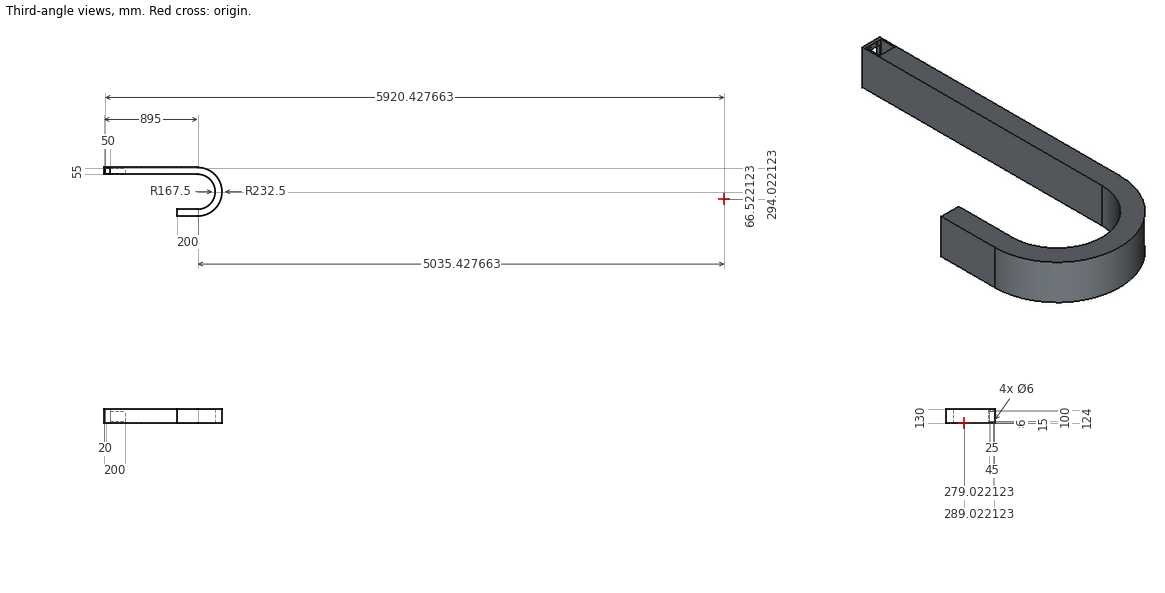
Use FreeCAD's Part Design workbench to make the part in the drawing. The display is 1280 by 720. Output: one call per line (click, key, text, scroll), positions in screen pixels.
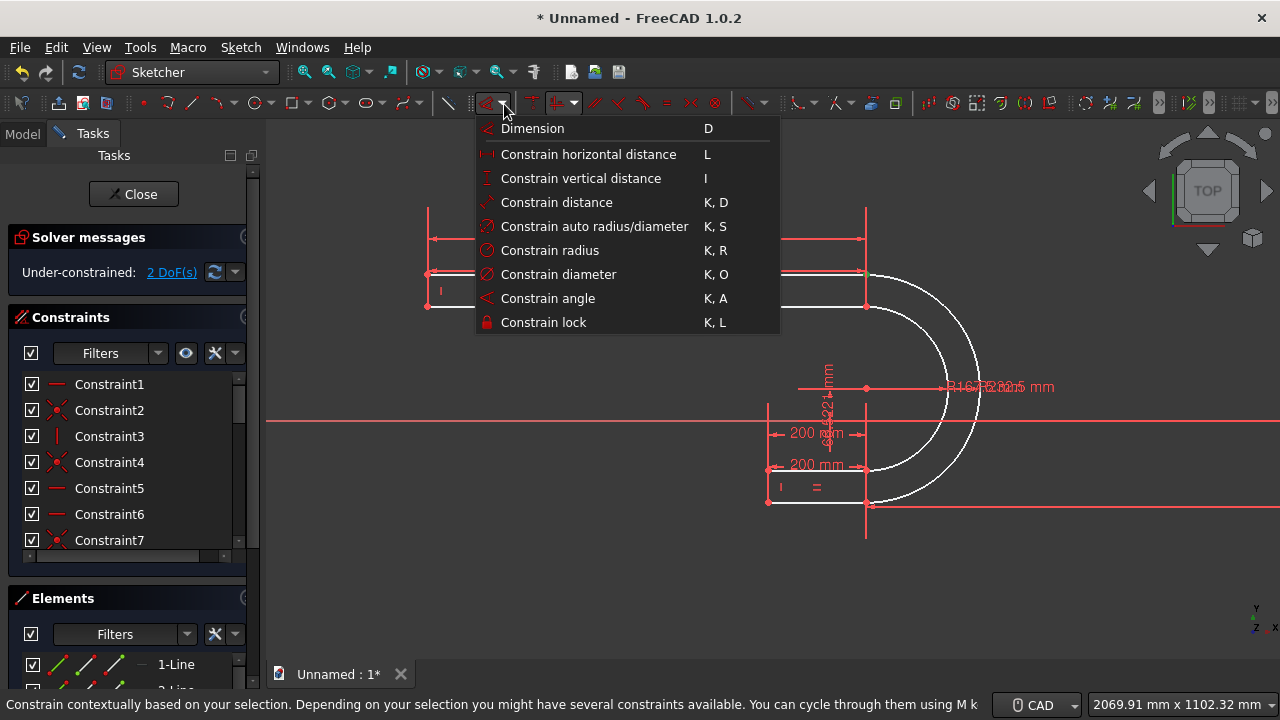
click(628, 154)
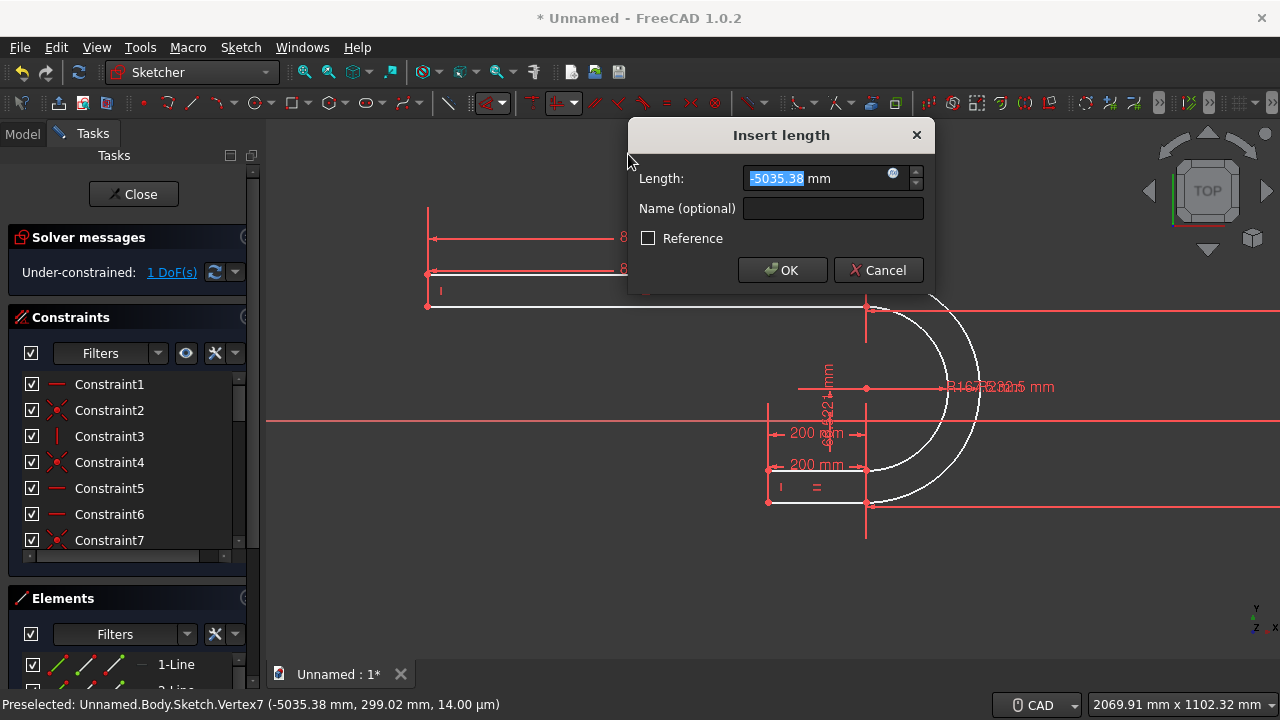
text(-5035.427663)
key(Return)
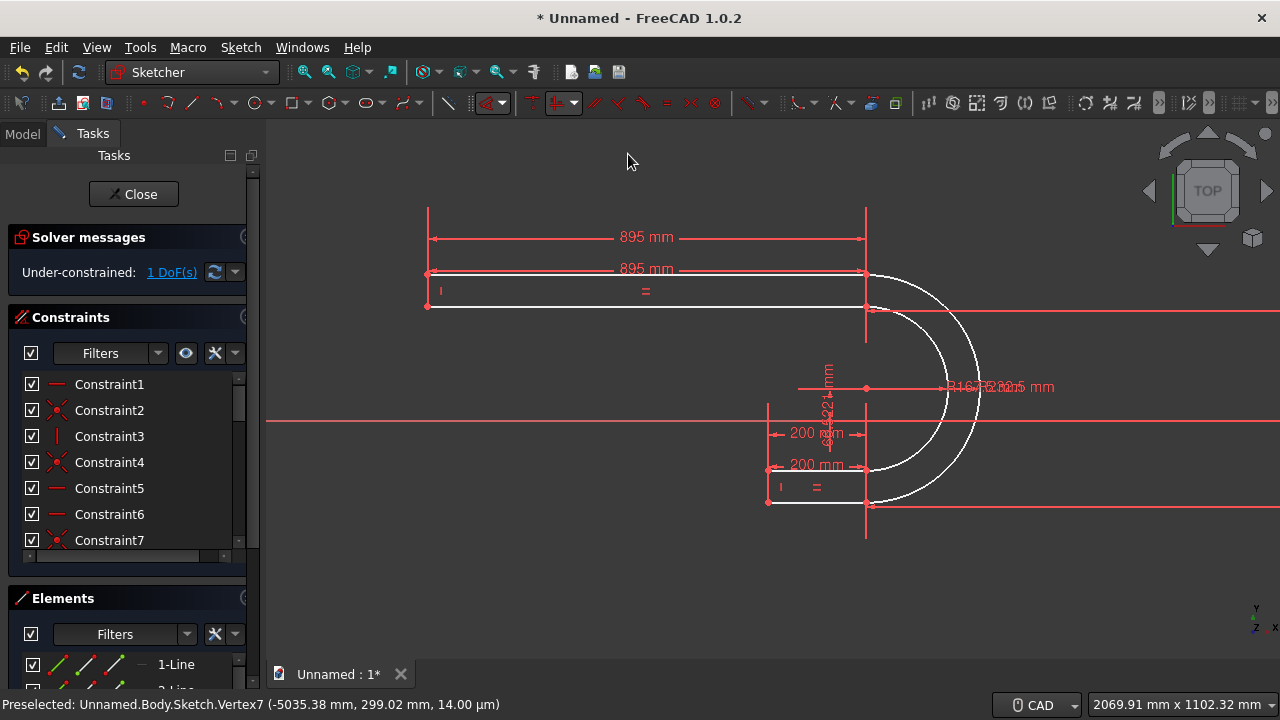
click(866, 389)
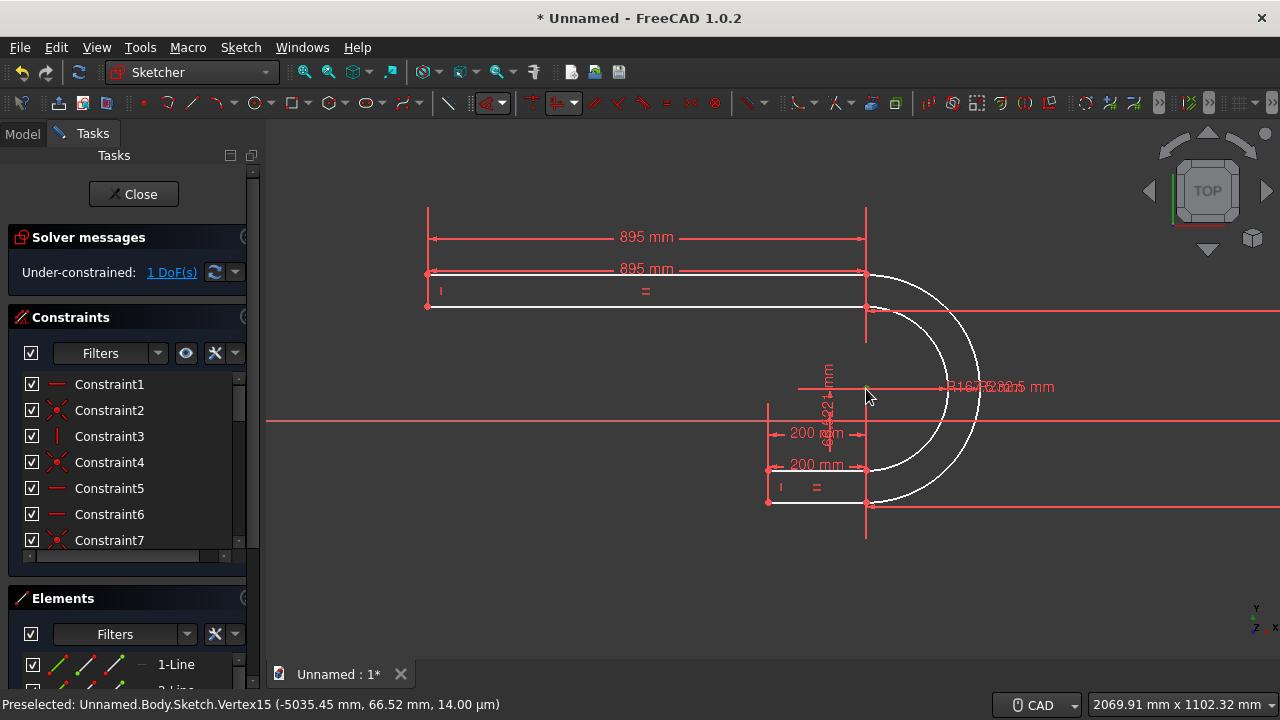
key(l)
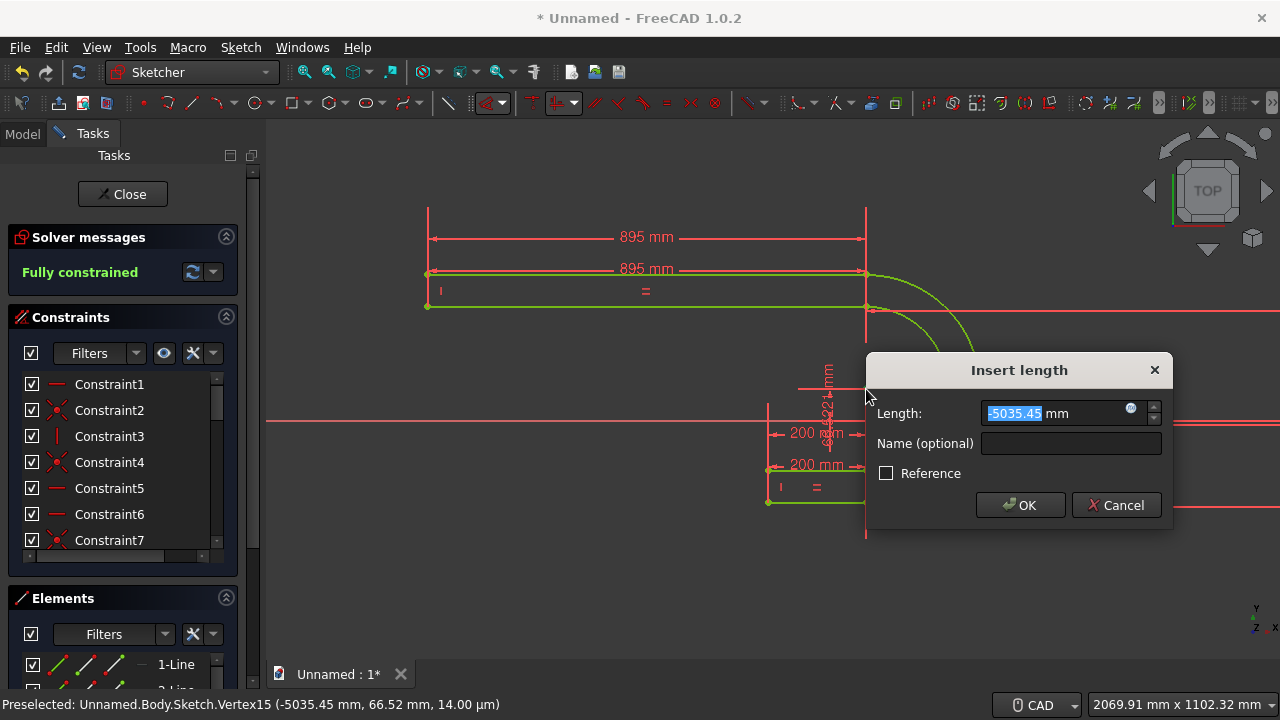
text(-5035.427663)
key(Return)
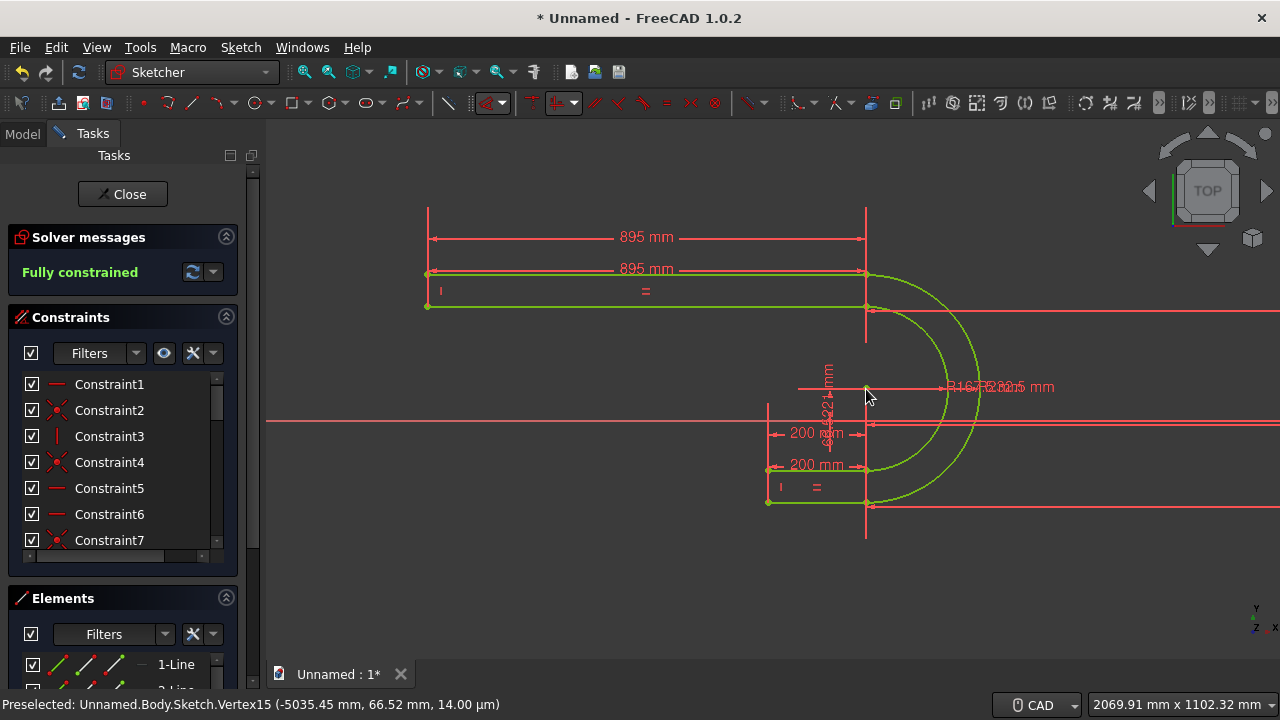
click(123, 194)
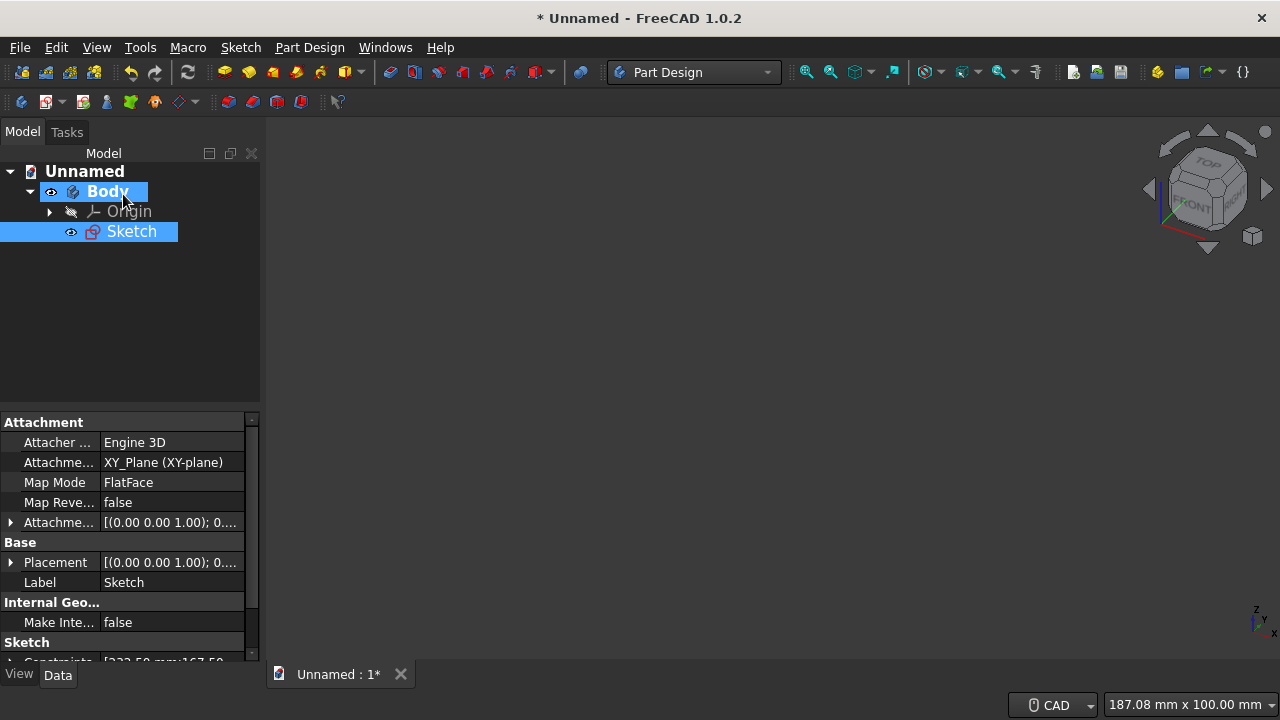
click(226, 72)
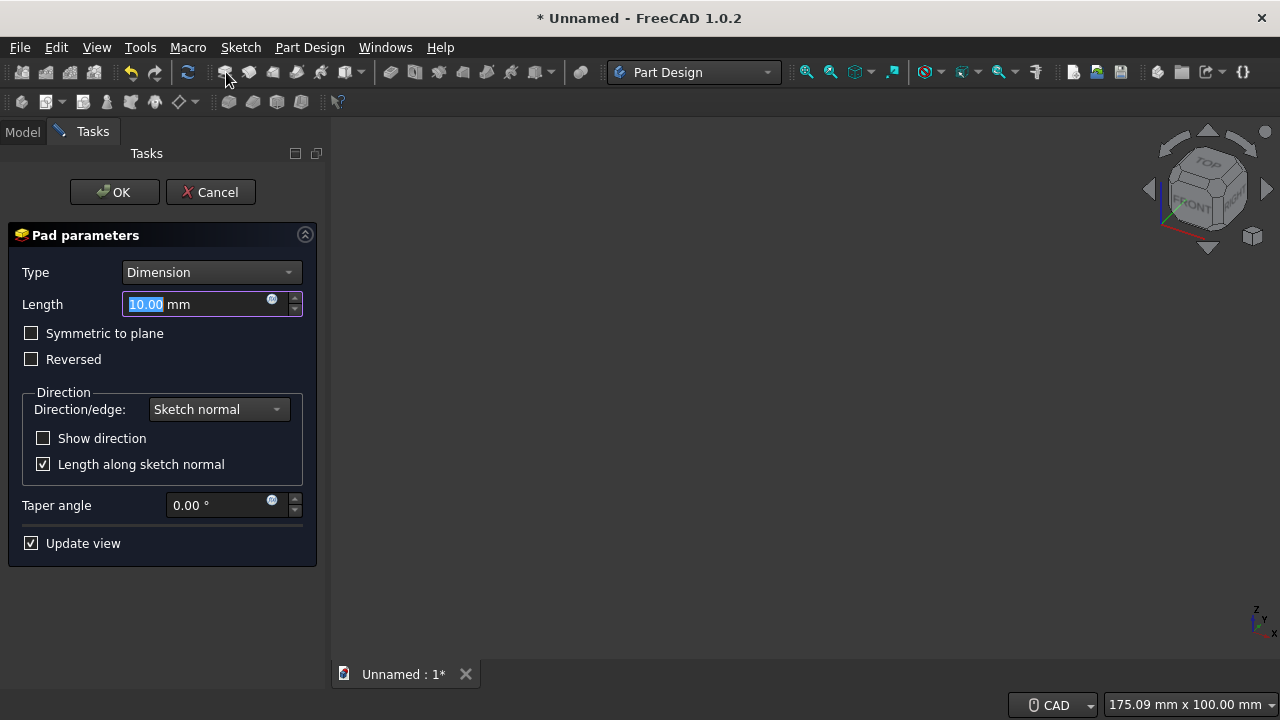
text(130)
key(Tab)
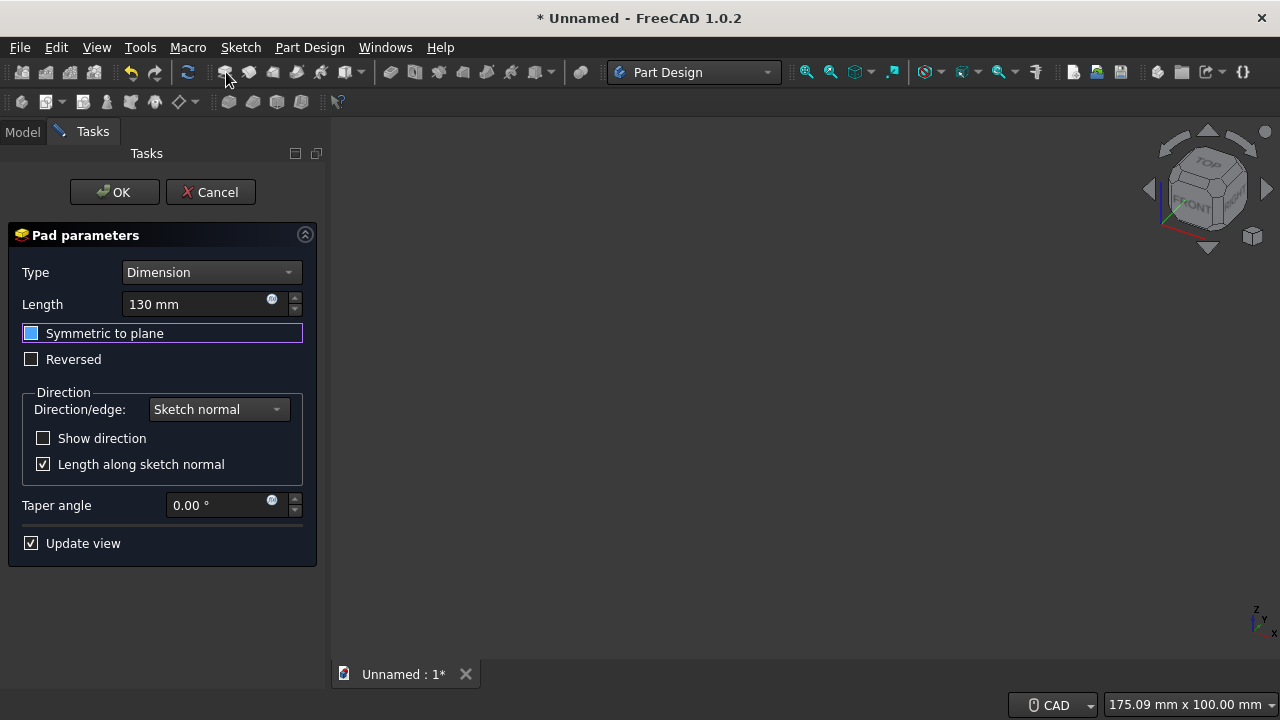
click(115, 192)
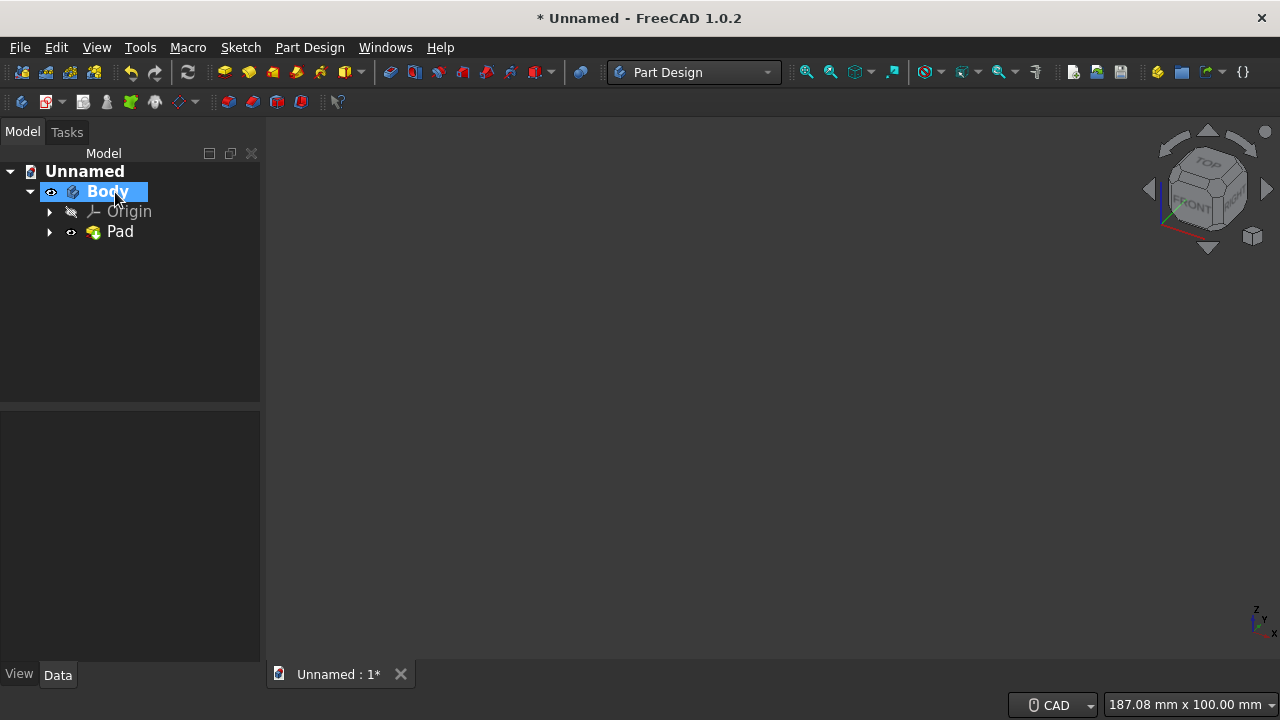
key(v)
key(f)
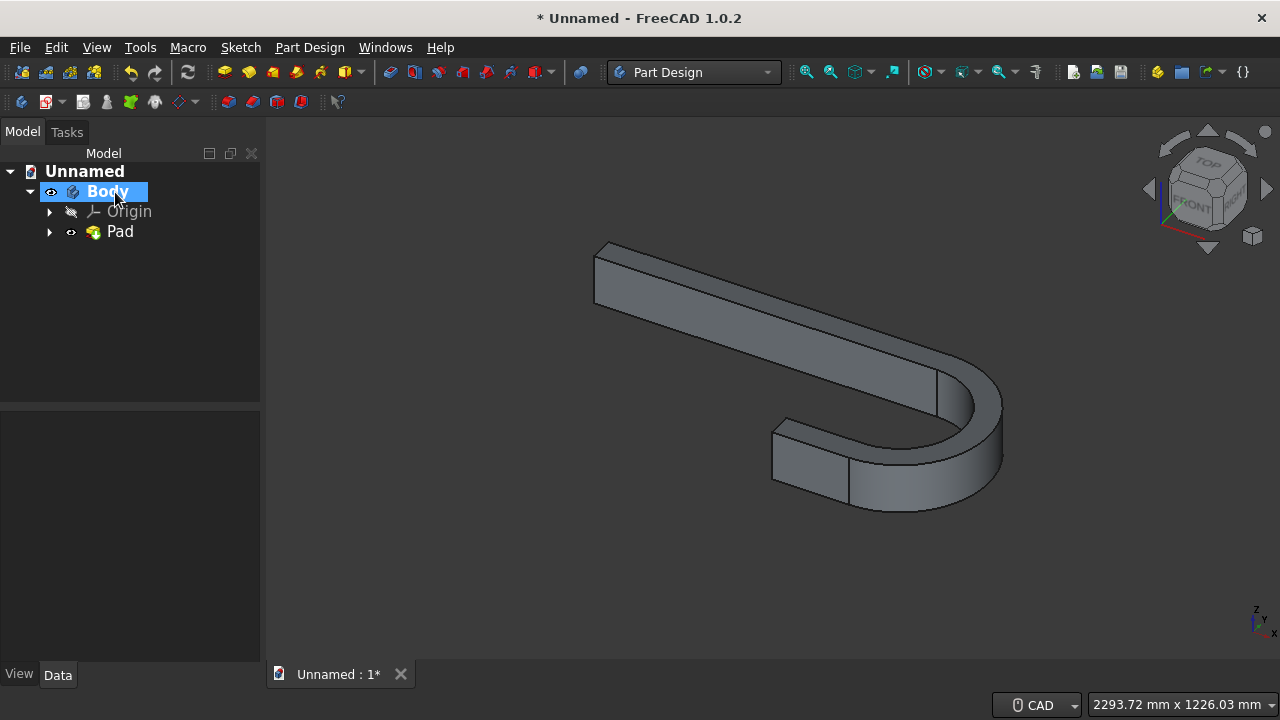
key(6)